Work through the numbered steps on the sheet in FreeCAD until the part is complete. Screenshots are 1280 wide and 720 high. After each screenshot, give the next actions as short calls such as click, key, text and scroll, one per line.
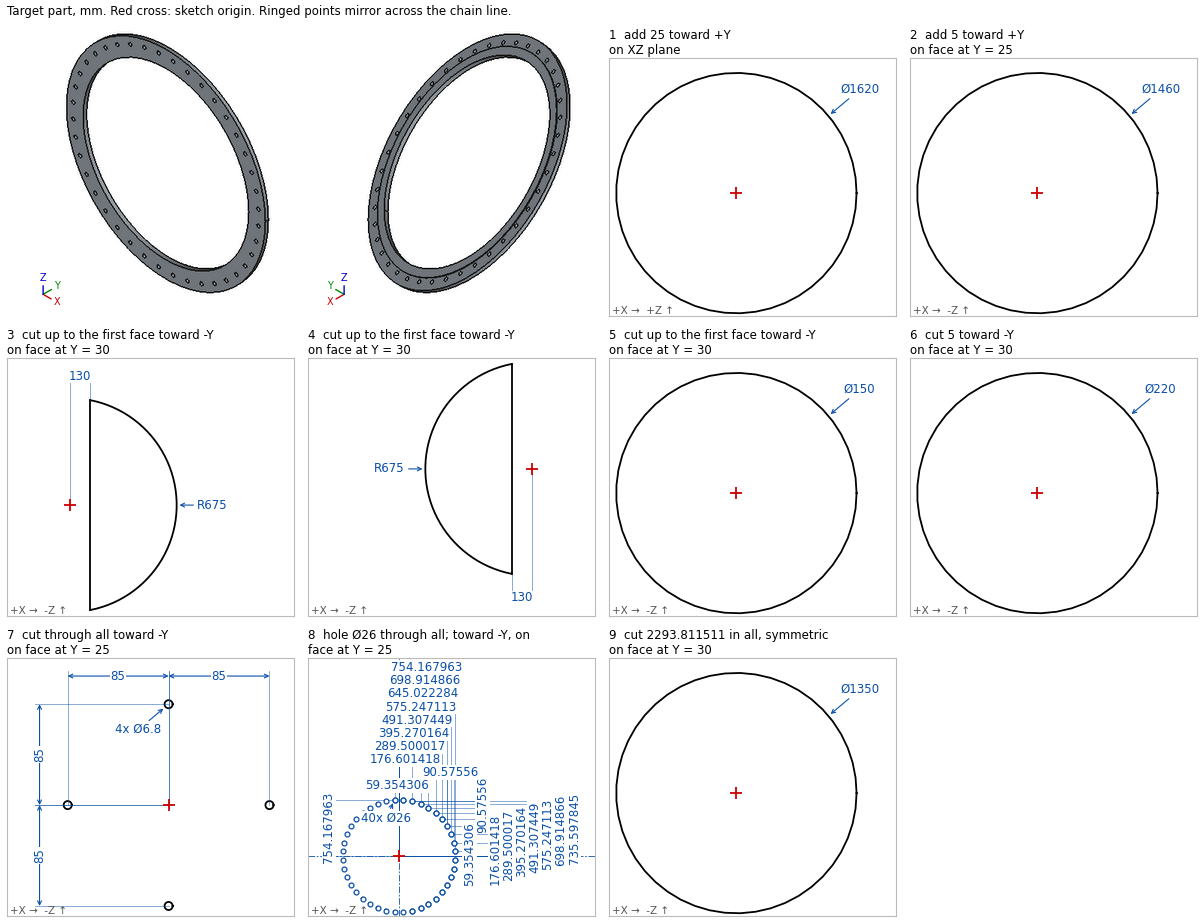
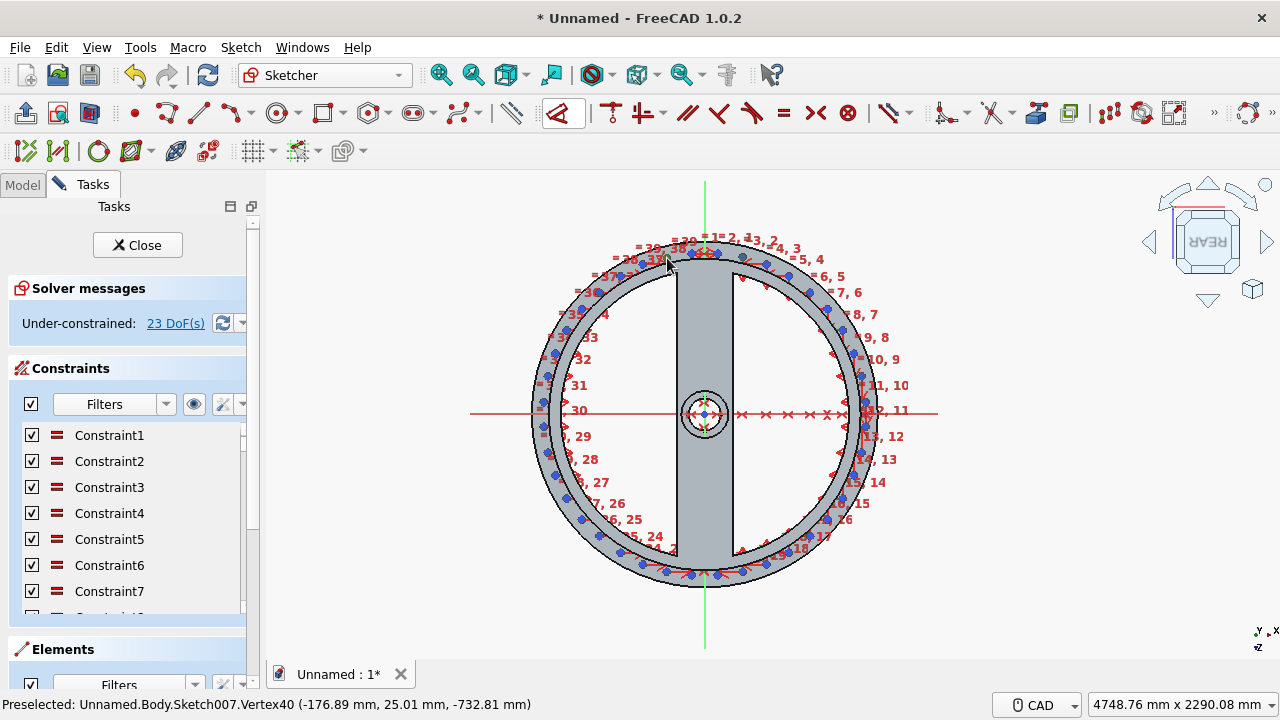
click(705, 507)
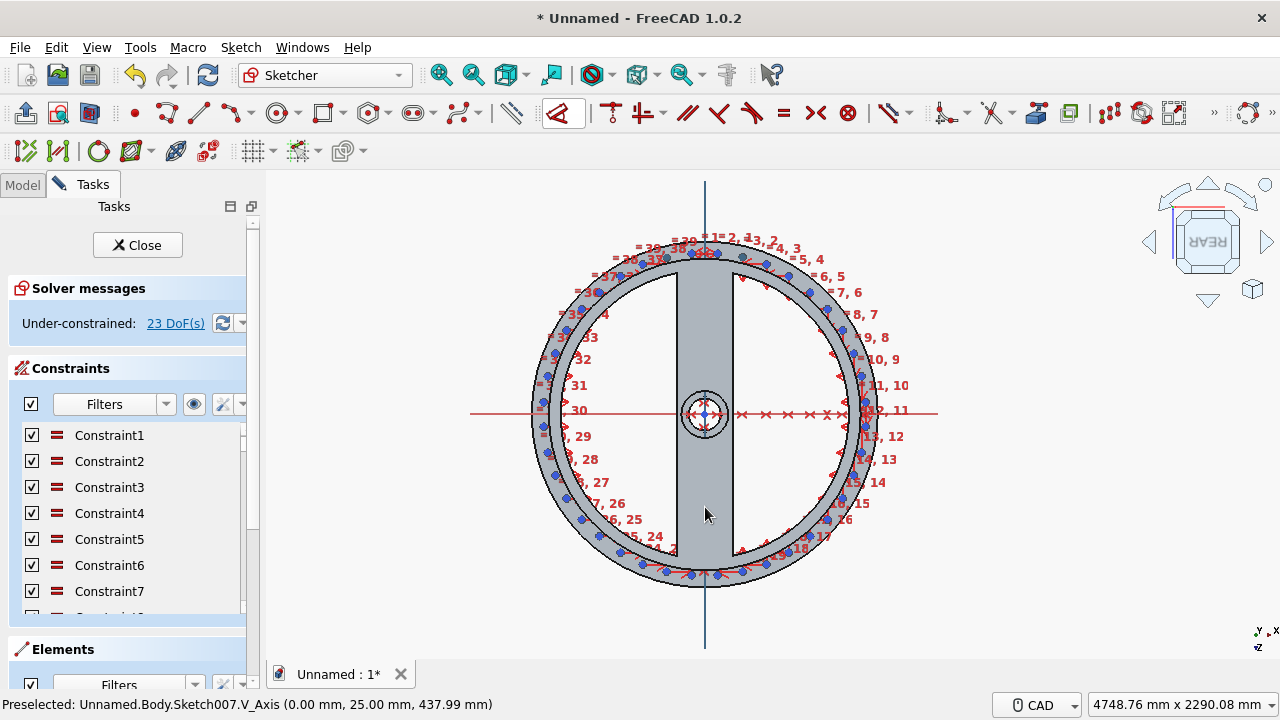
click(816, 114)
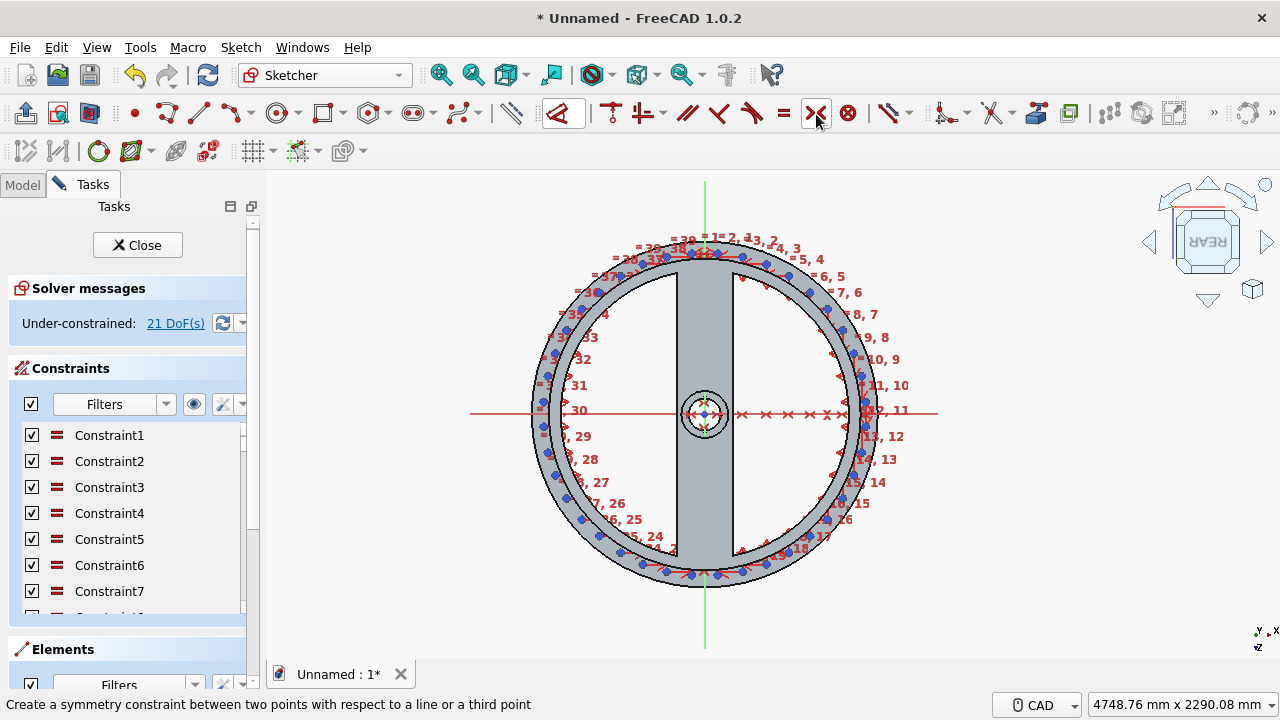
scroll(694, 251, up, 10)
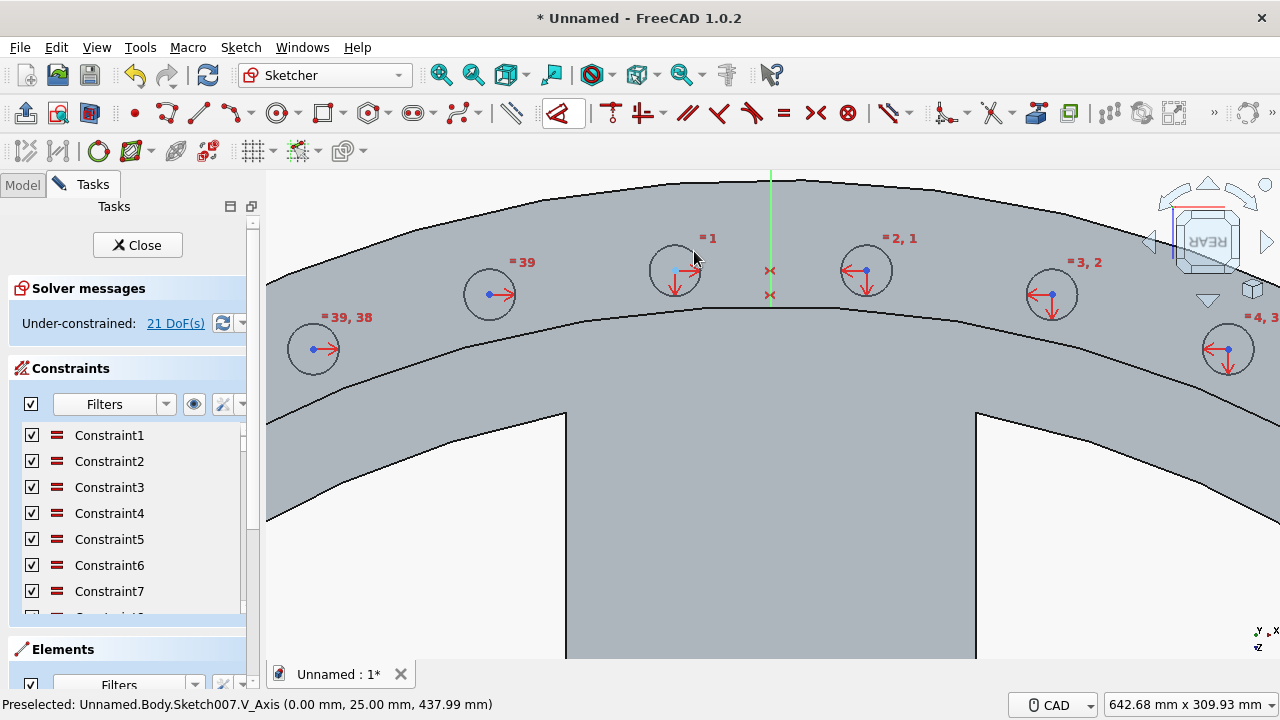
click(693, 253)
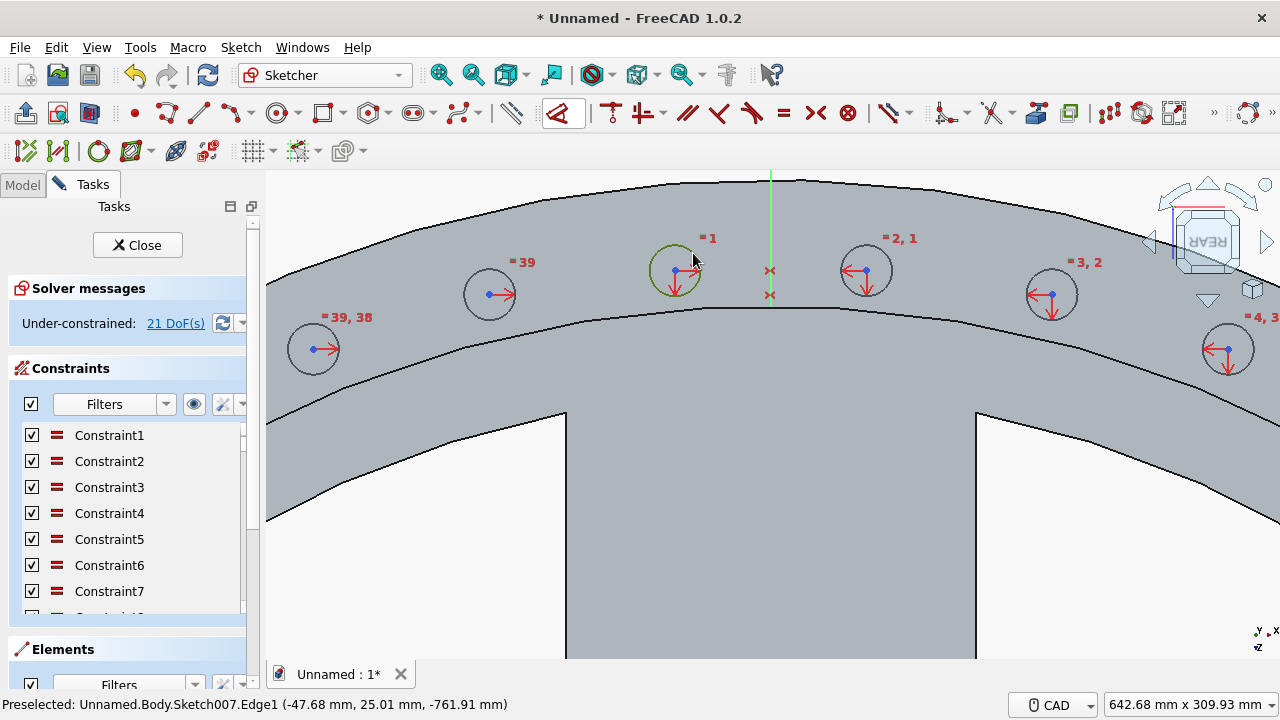
key(k)
key(o)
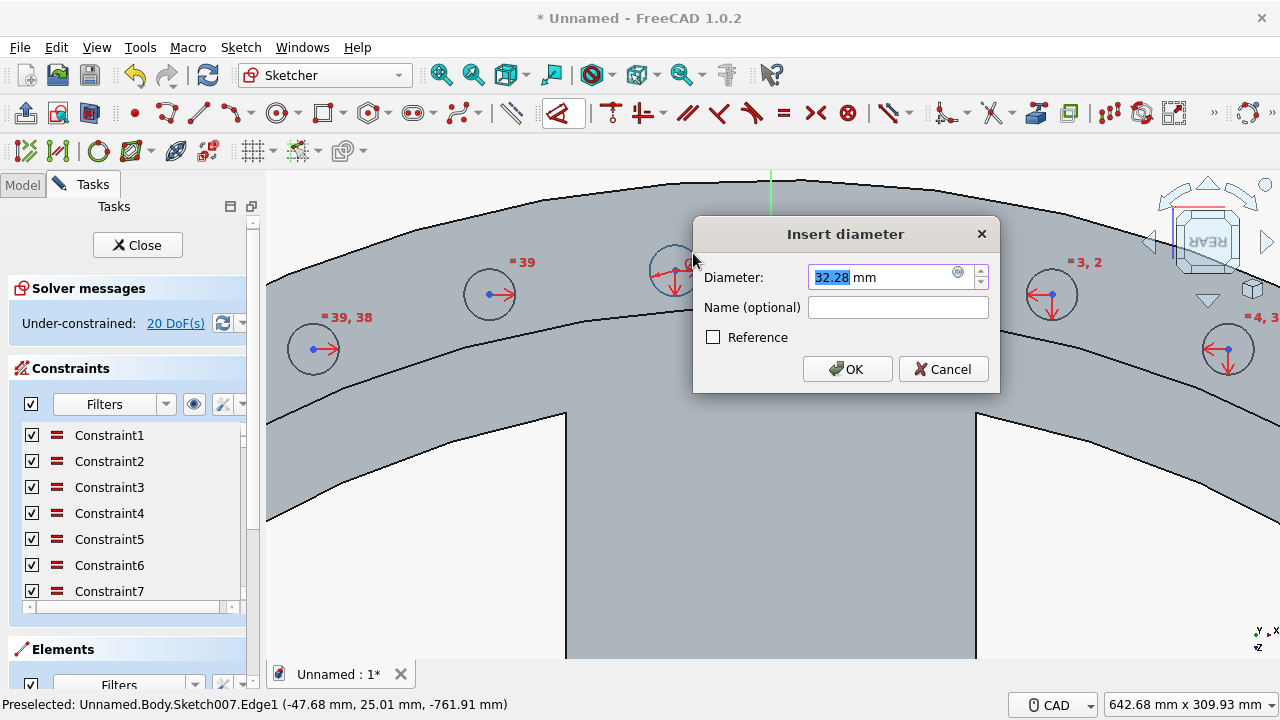
text(26)
key(Return)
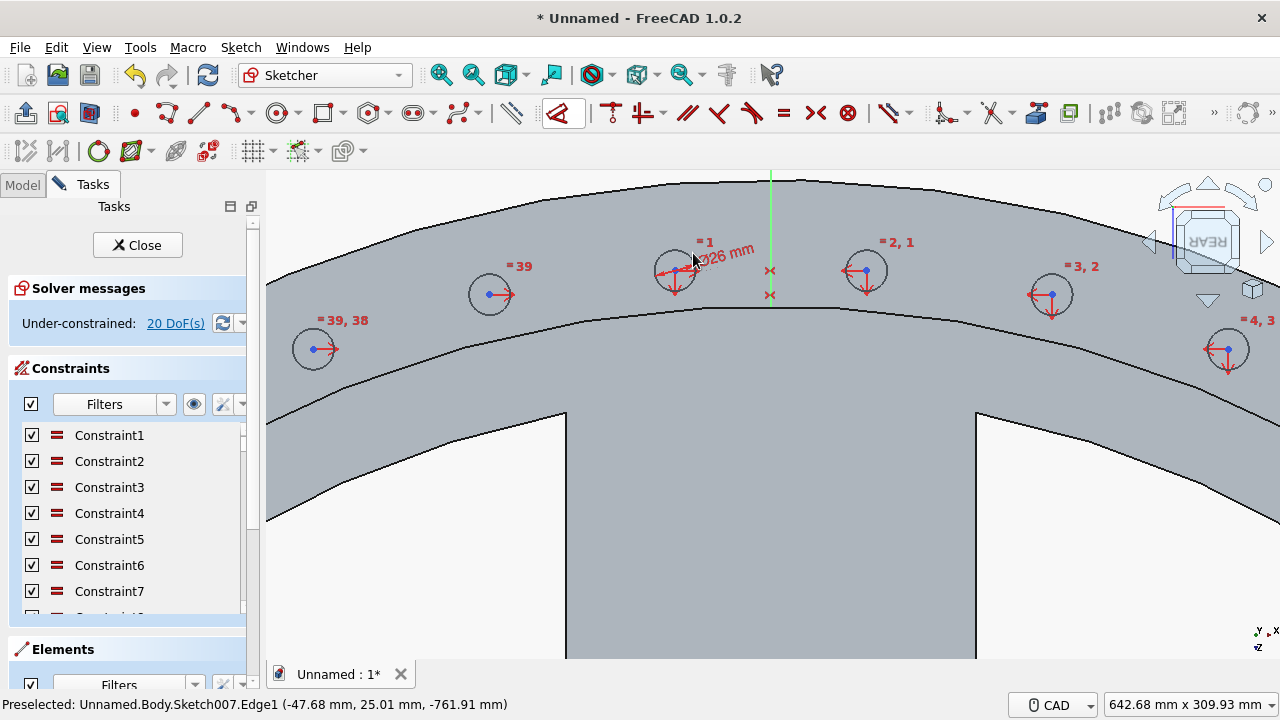
click(675, 271)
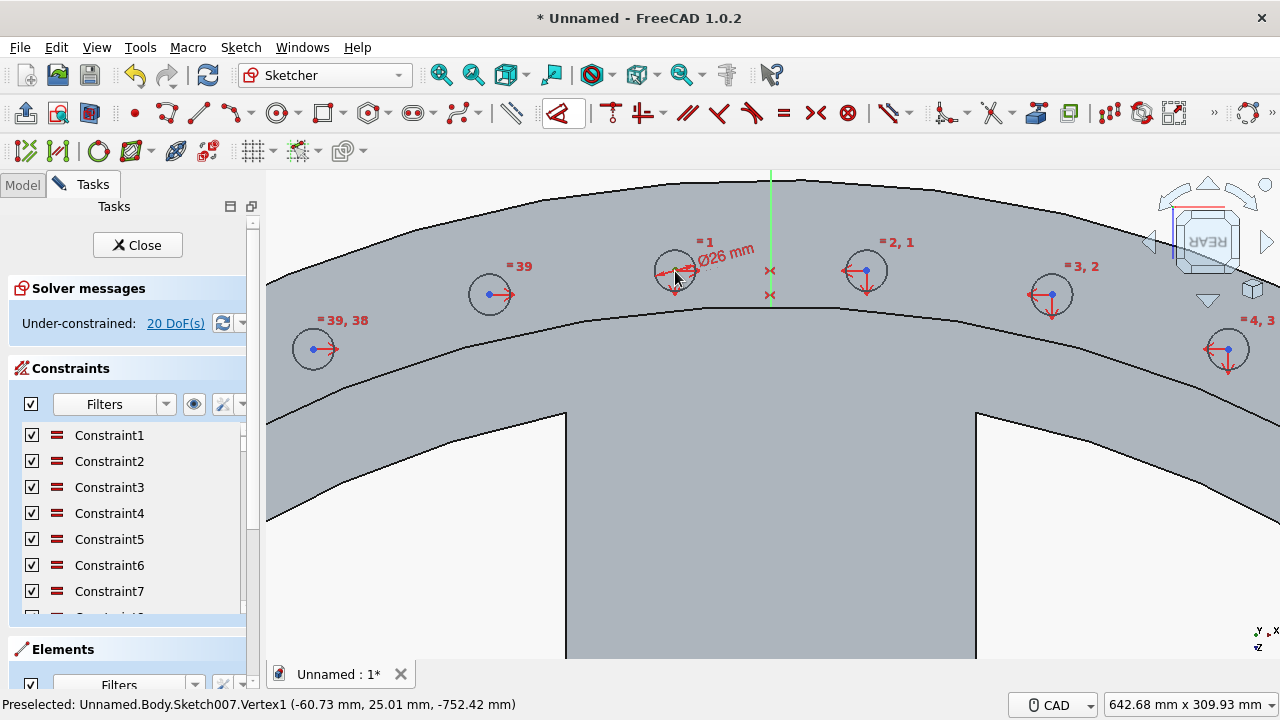
key(l)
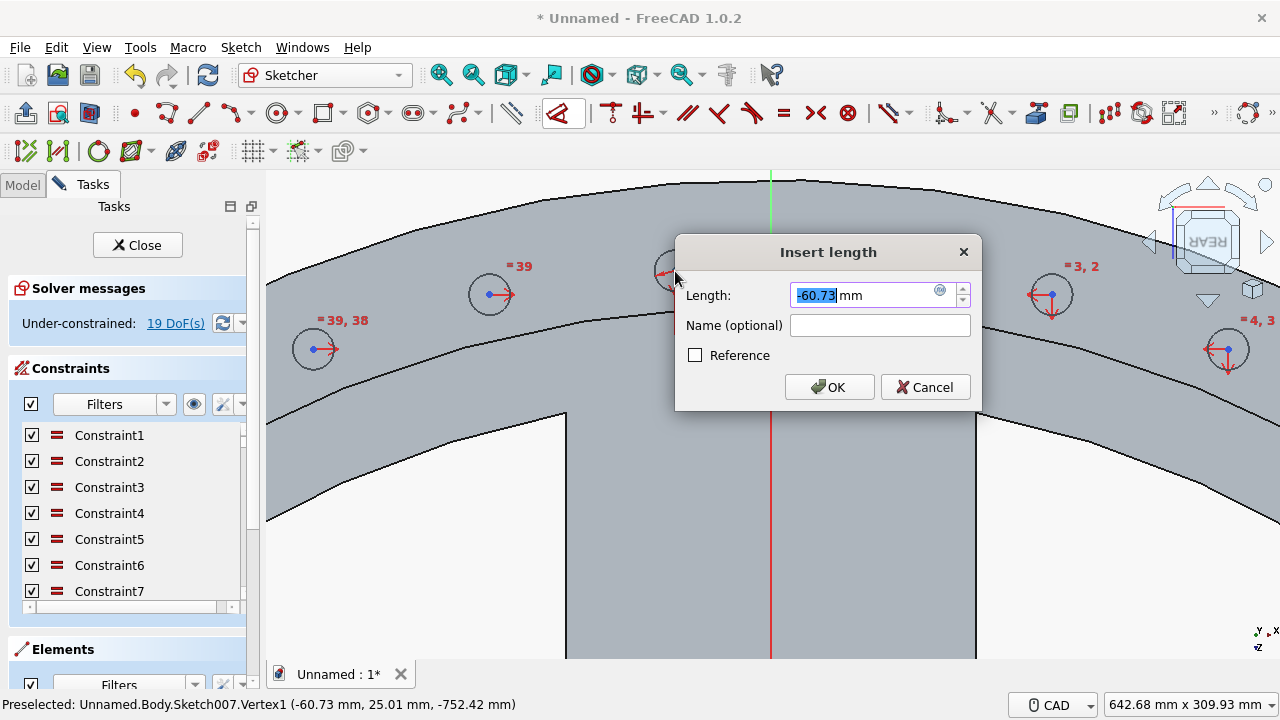
text(-59.354306)
key(Return)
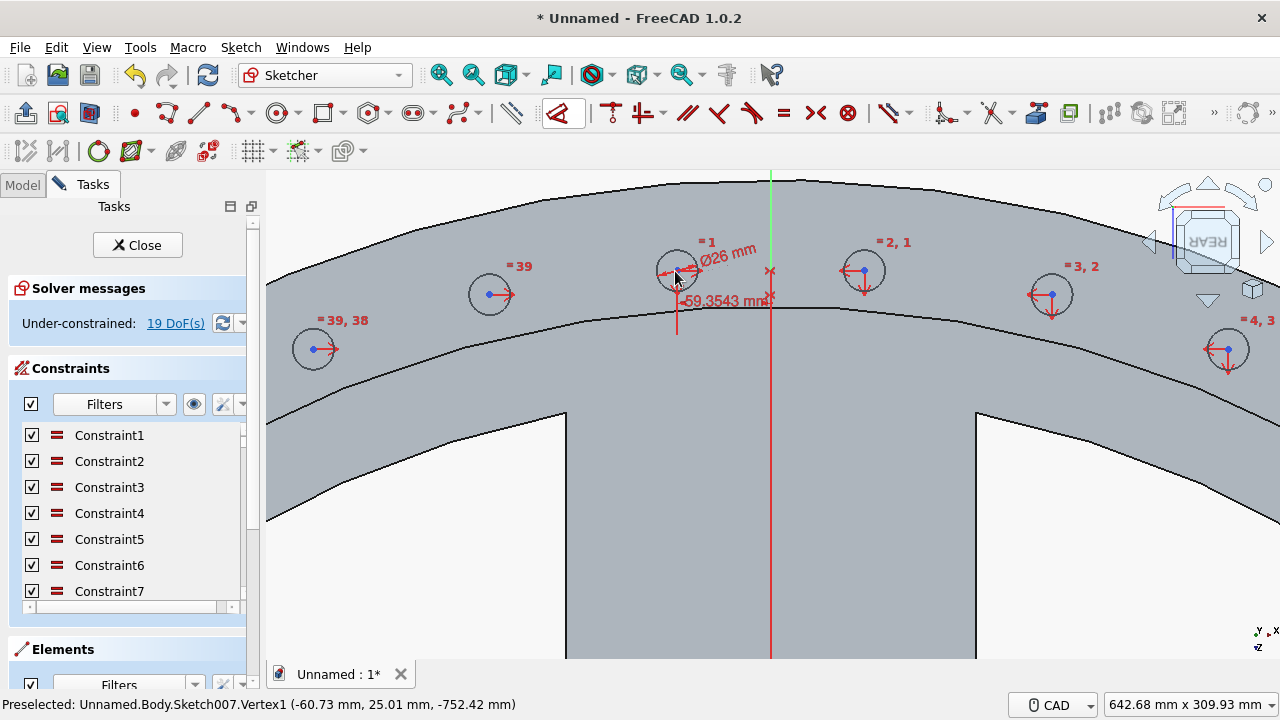
scroll(694, 251, down, 10)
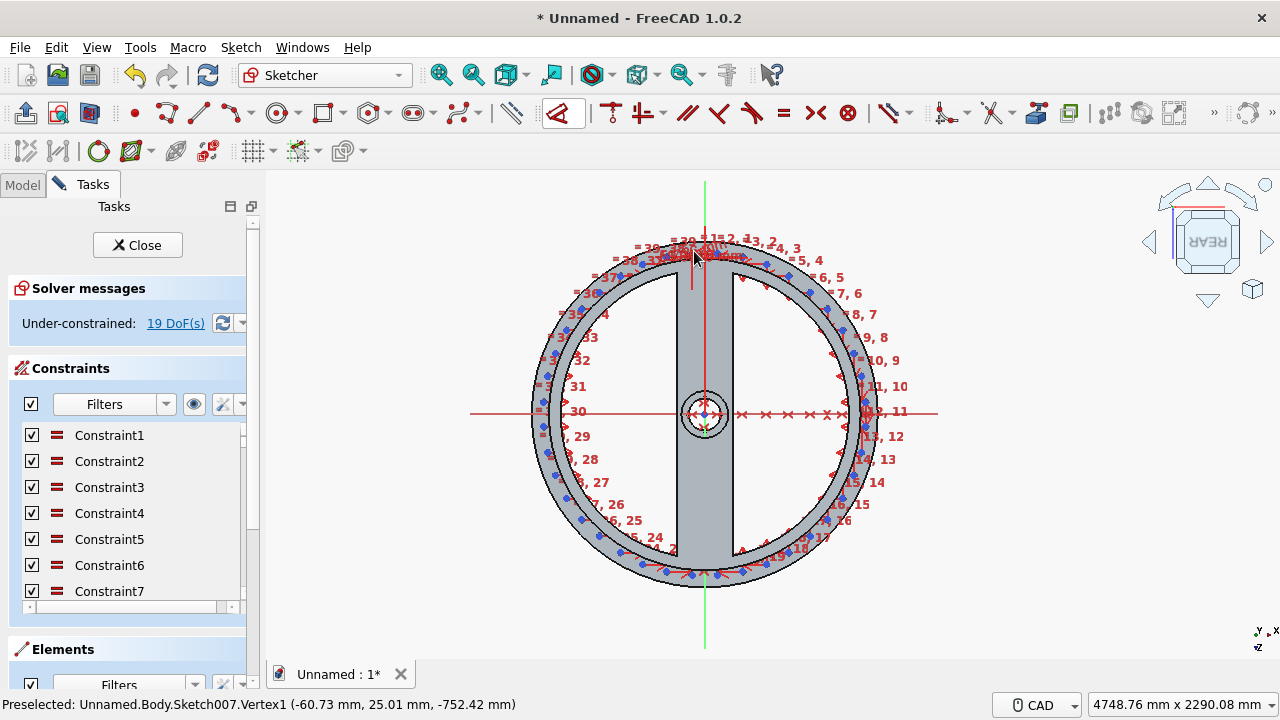
scroll(866, 402, up, 6)